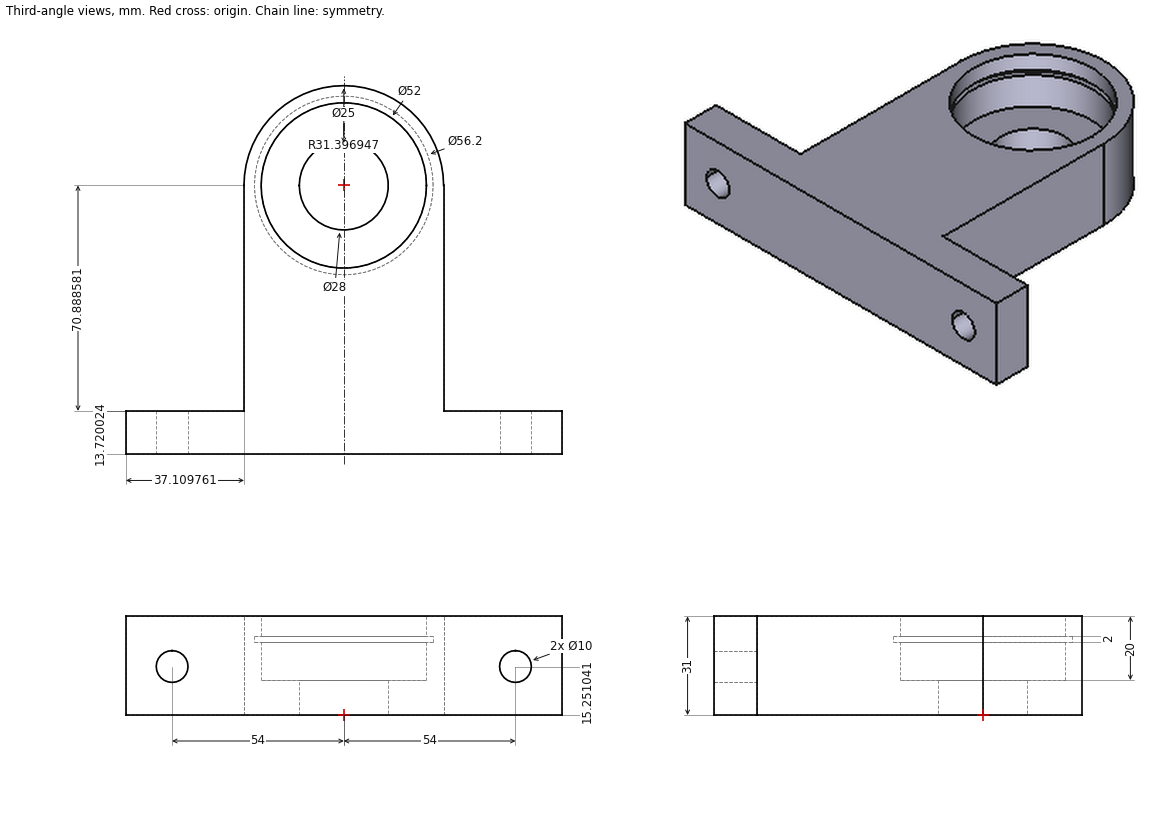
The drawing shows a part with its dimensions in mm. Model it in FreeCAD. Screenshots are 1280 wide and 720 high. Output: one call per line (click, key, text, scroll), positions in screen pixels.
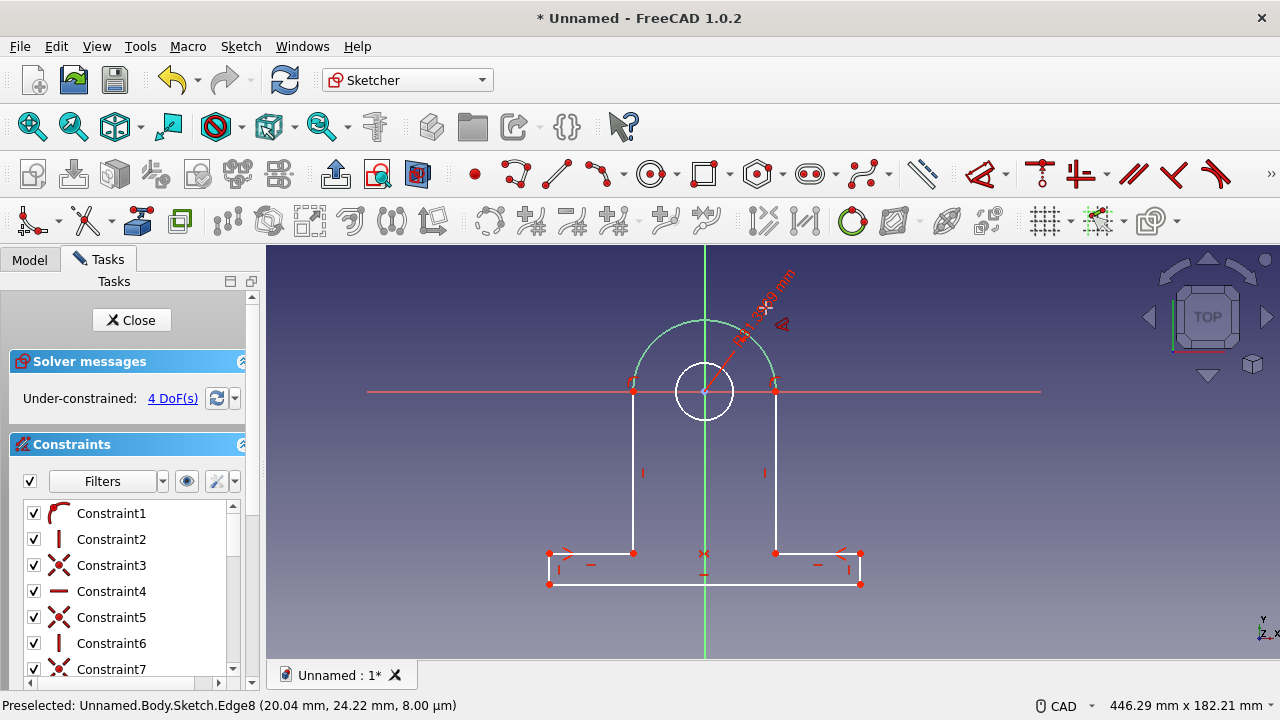
click(725, 371)
click(748, 435)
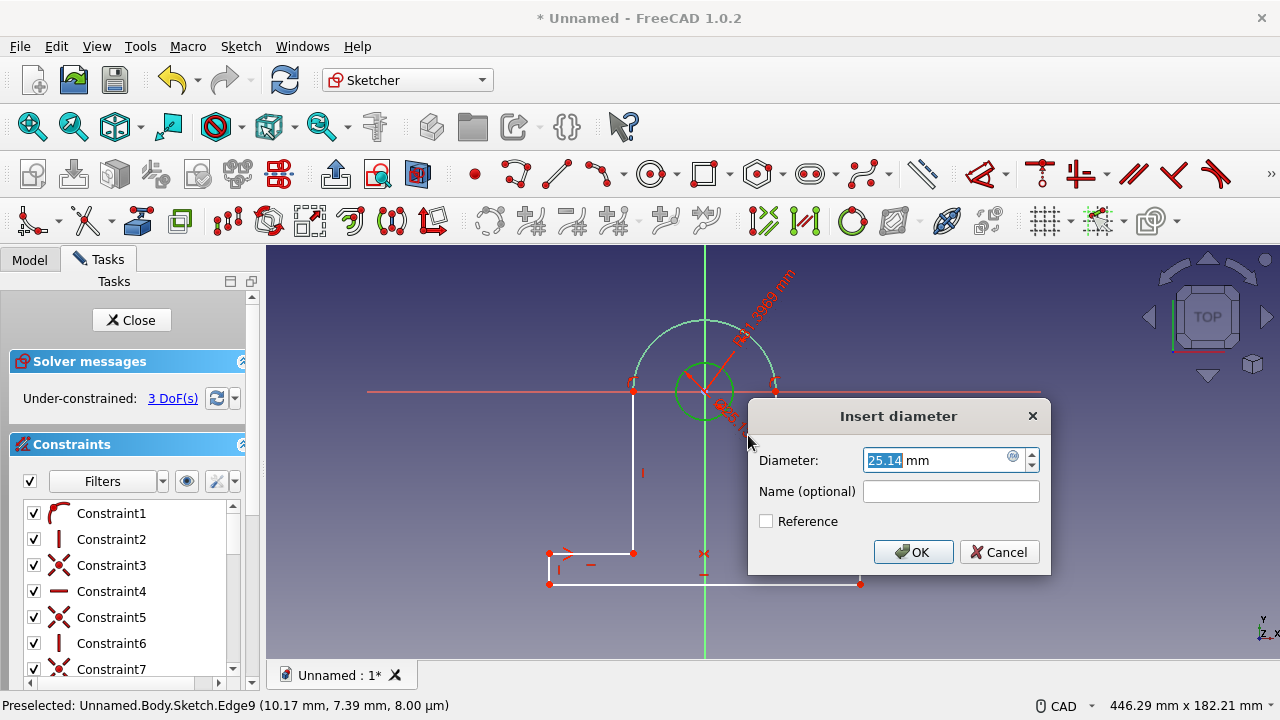
text(25)
key(Return)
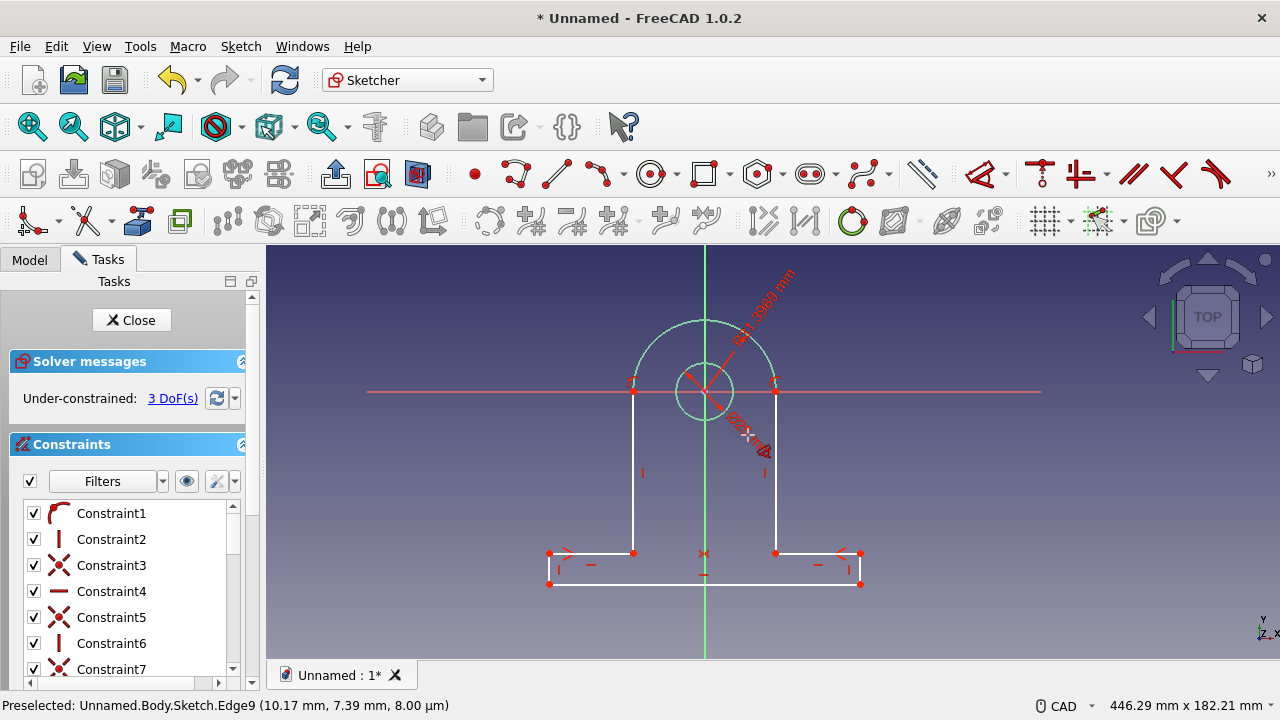
click(633, 440)
click(599, 473)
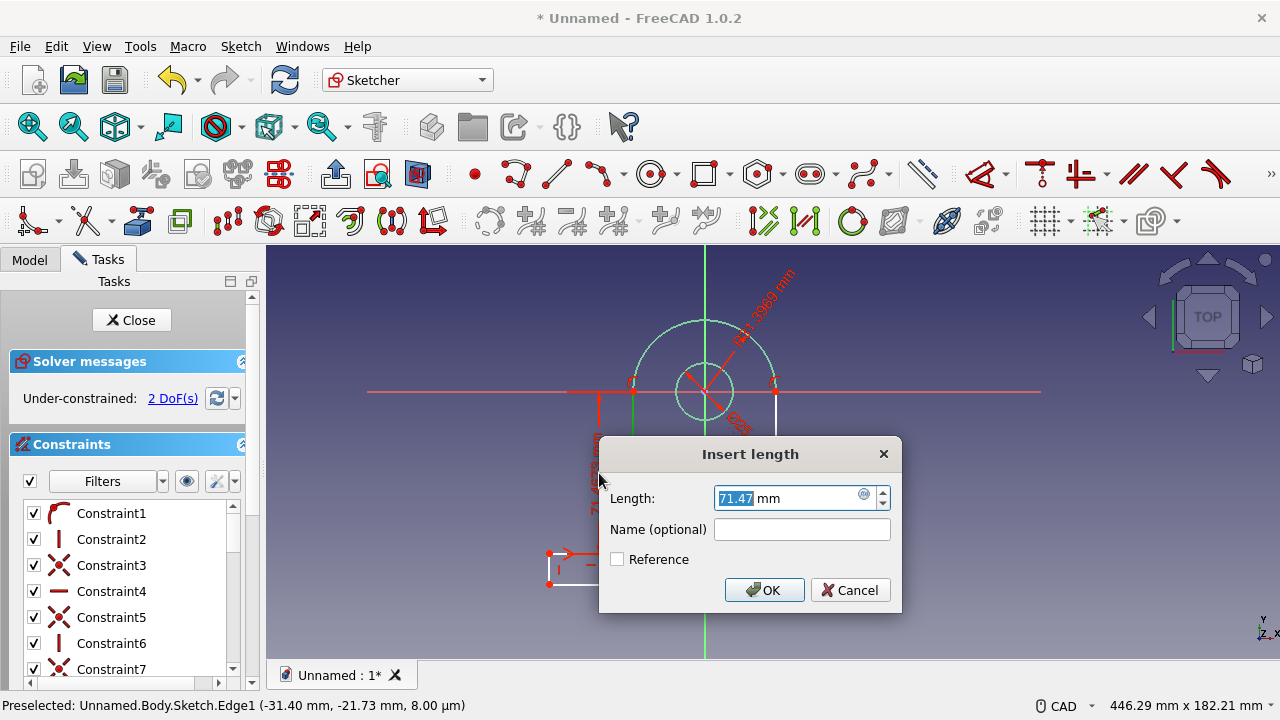
text(70.888581)
key(Return)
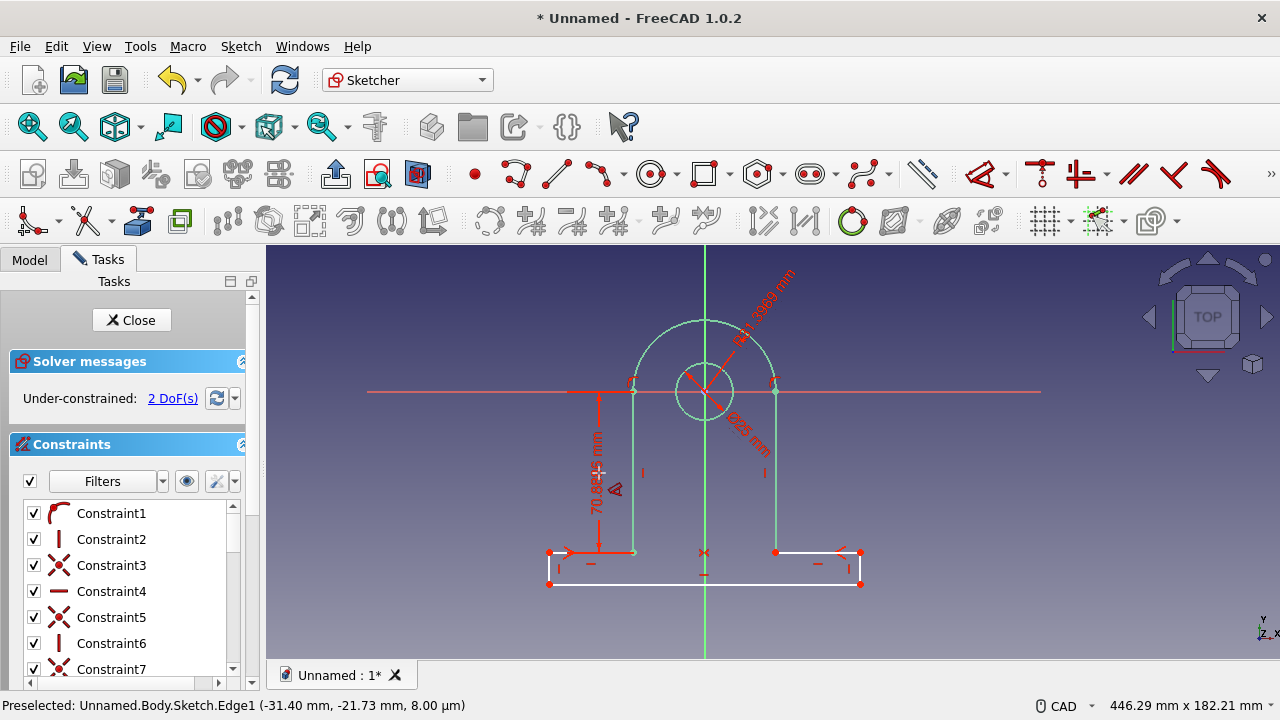
click(608, 553)
click(591, 519)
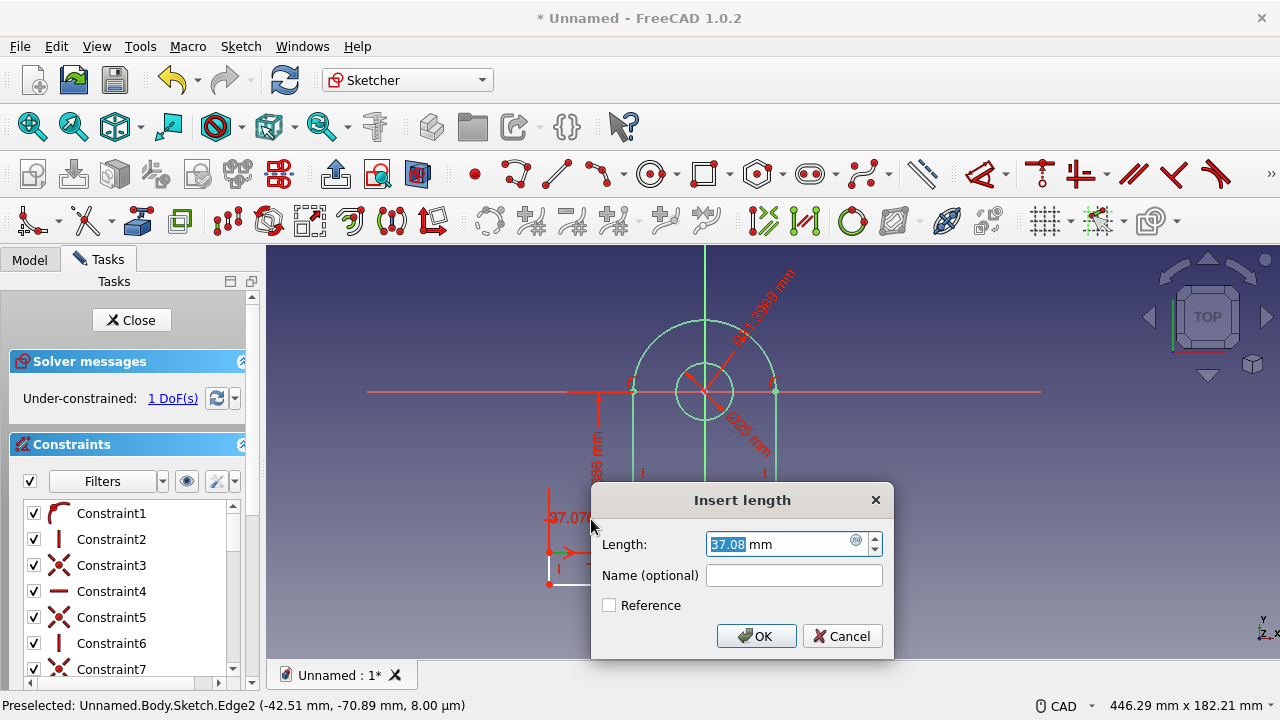
text(37.109761)
key(Return)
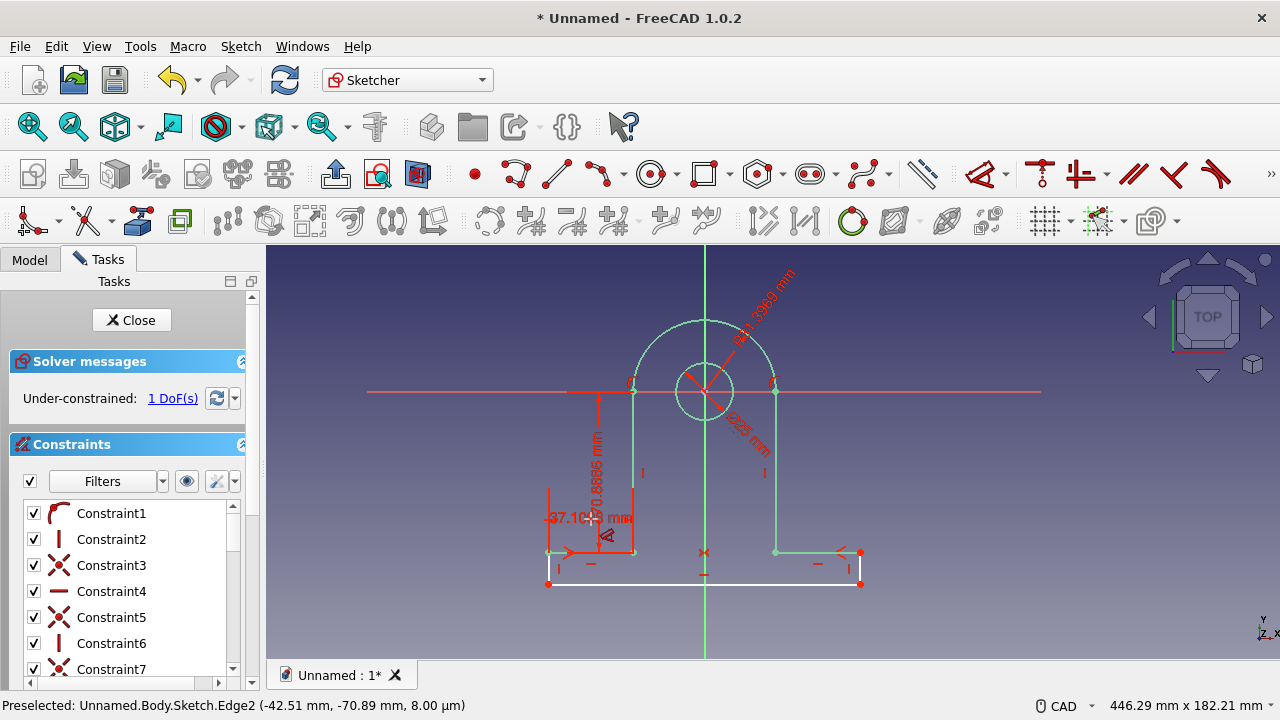
scroll(549, 562, up, 2)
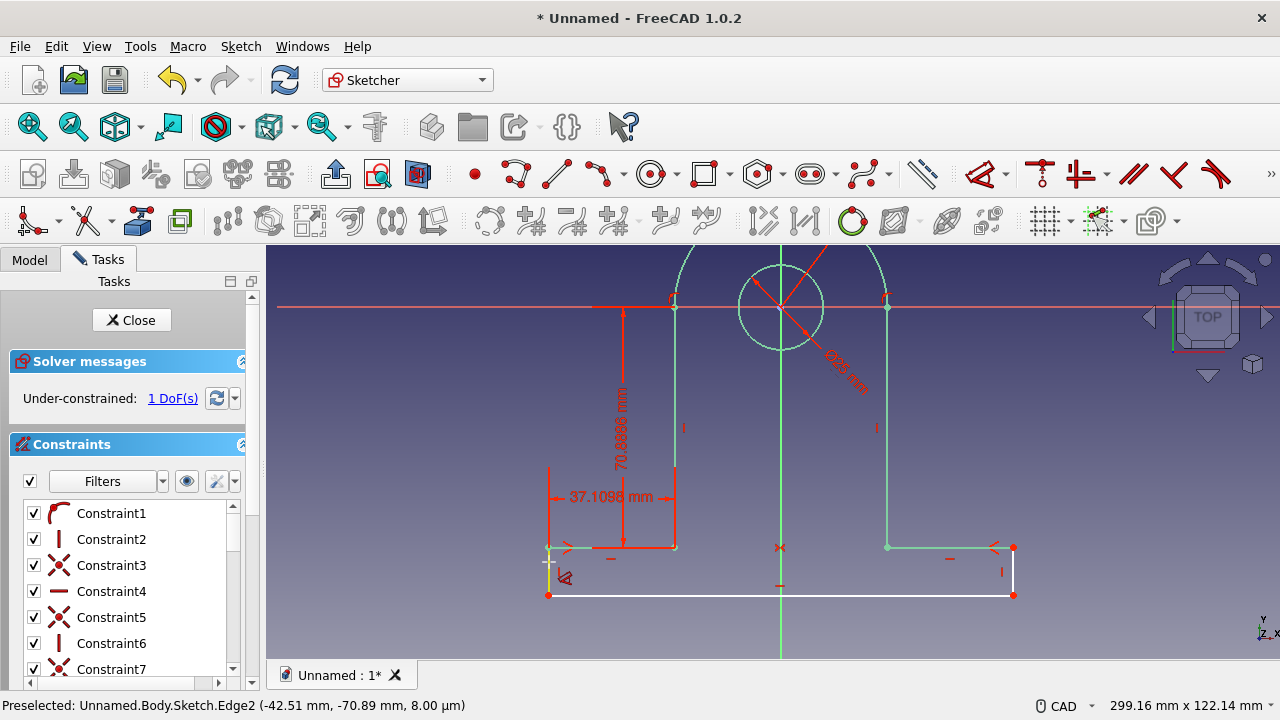
click(549, 562)
click(515, 572)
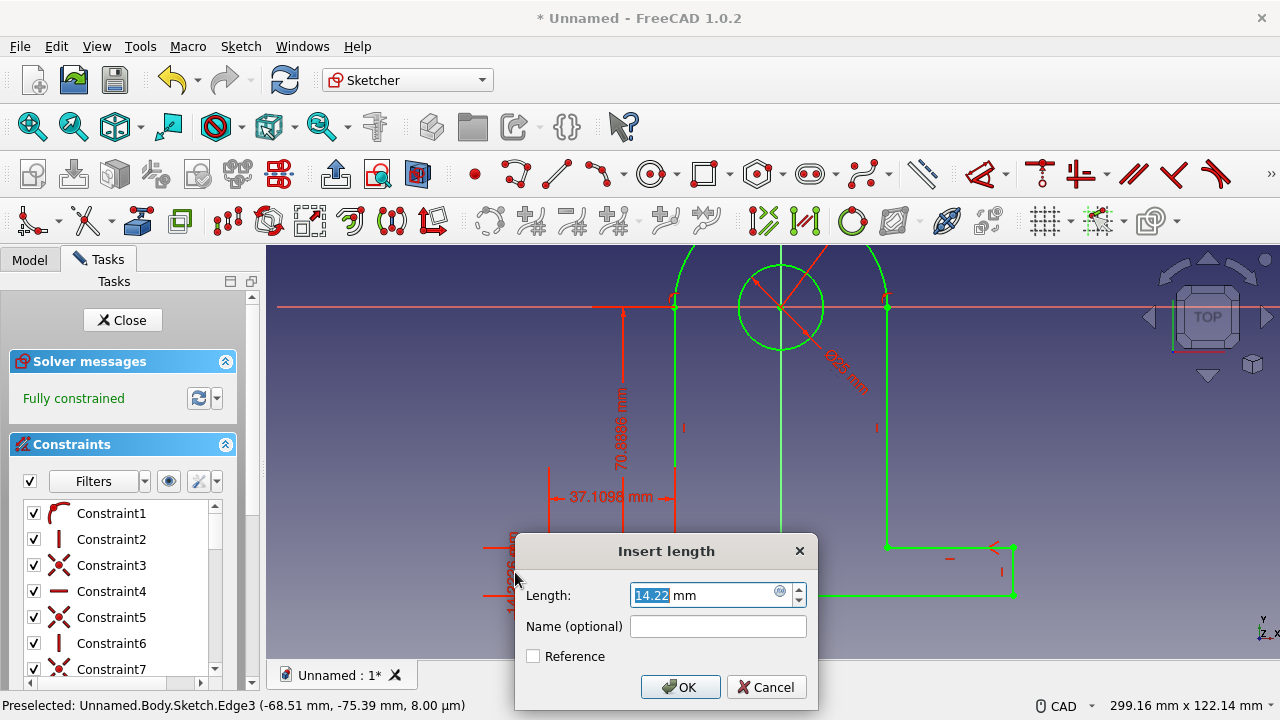
text(13.720024)
key(Return)
key(Escape)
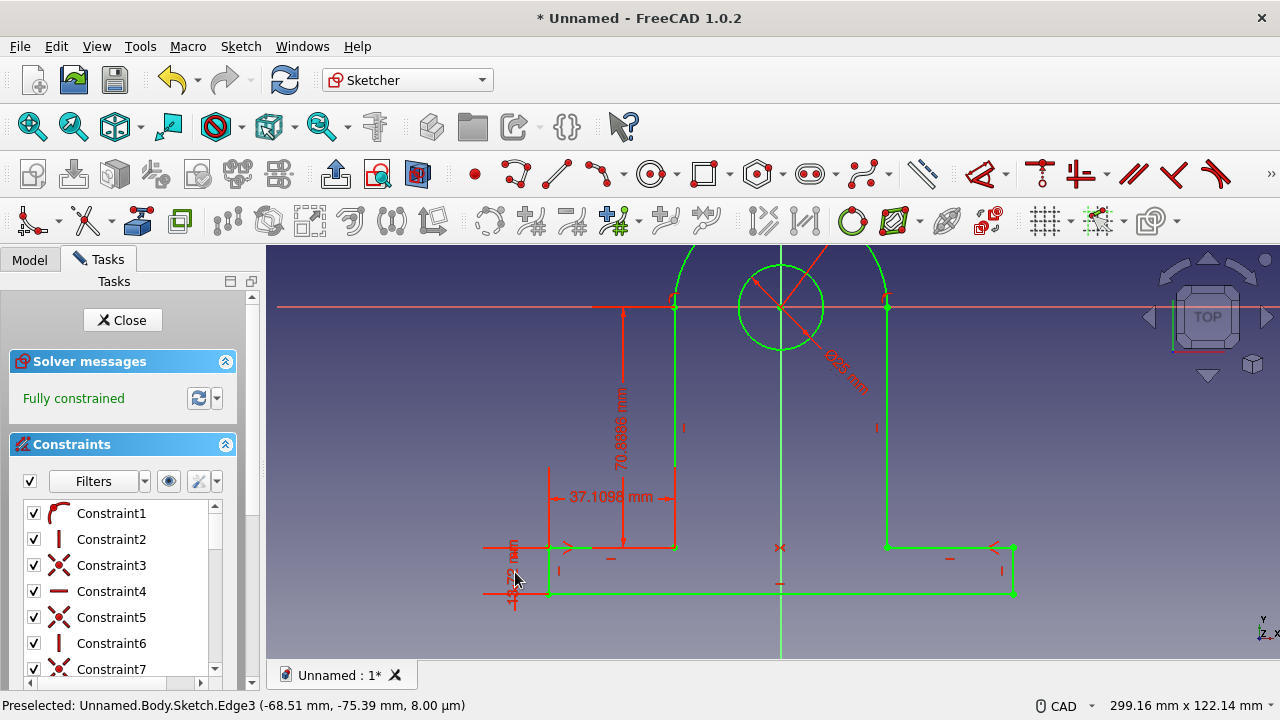
click(123, 320)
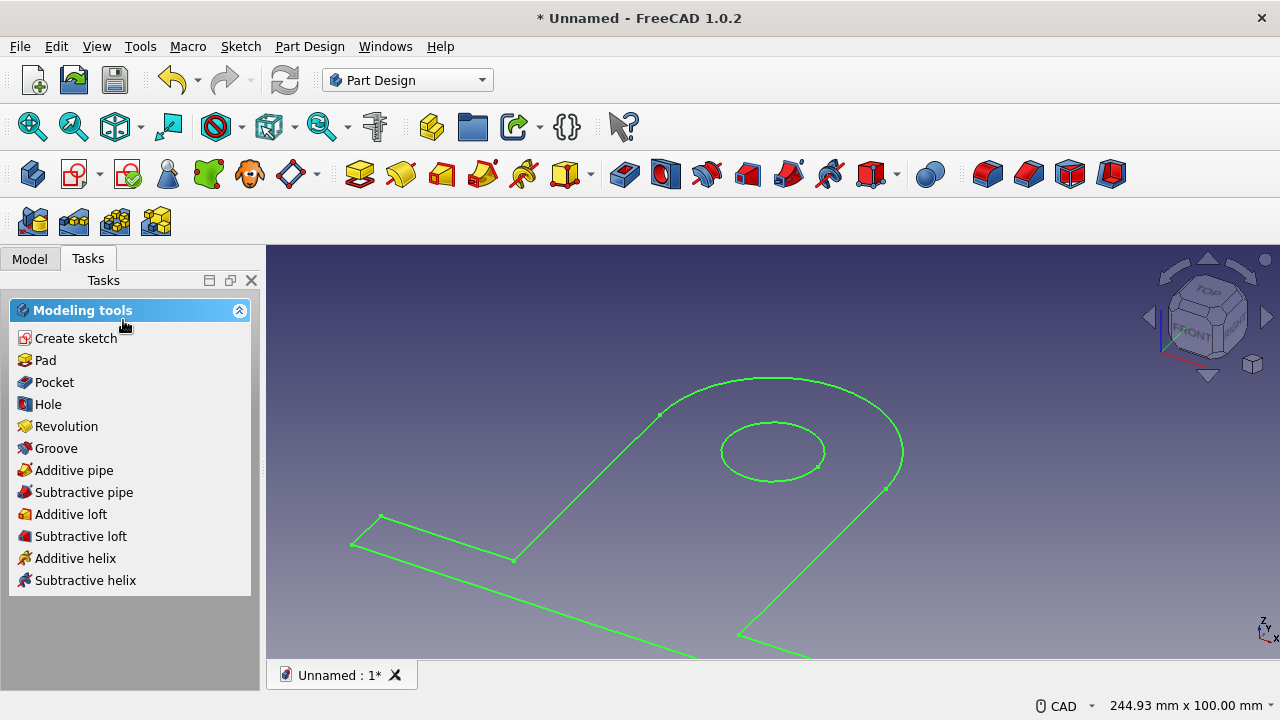
click(360, 174)